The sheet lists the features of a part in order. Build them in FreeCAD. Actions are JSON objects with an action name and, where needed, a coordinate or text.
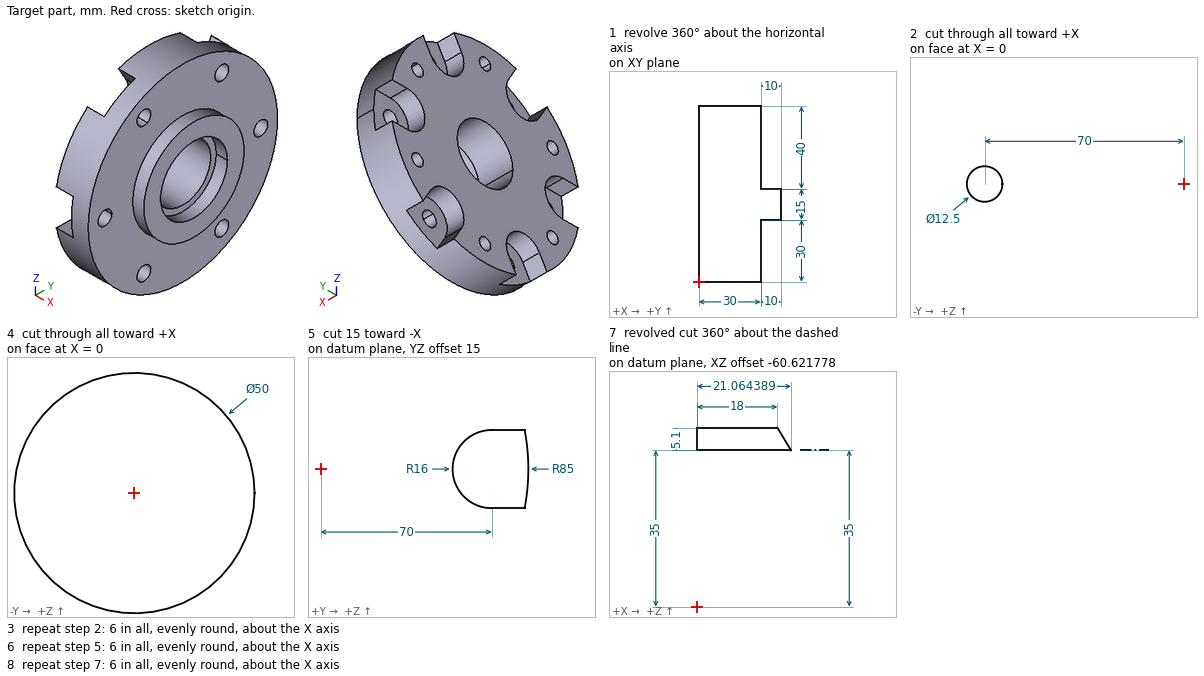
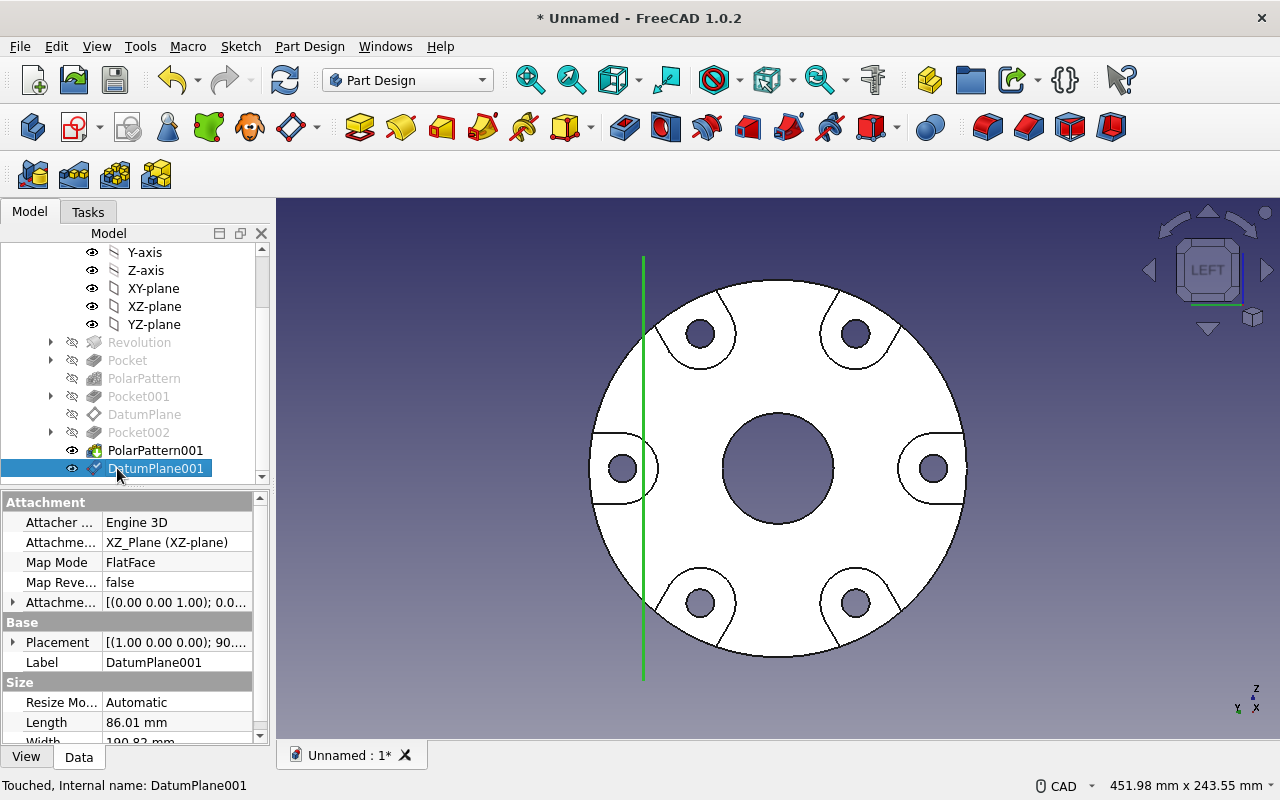
{"action": "left_click", "coordinate": [74, 128]}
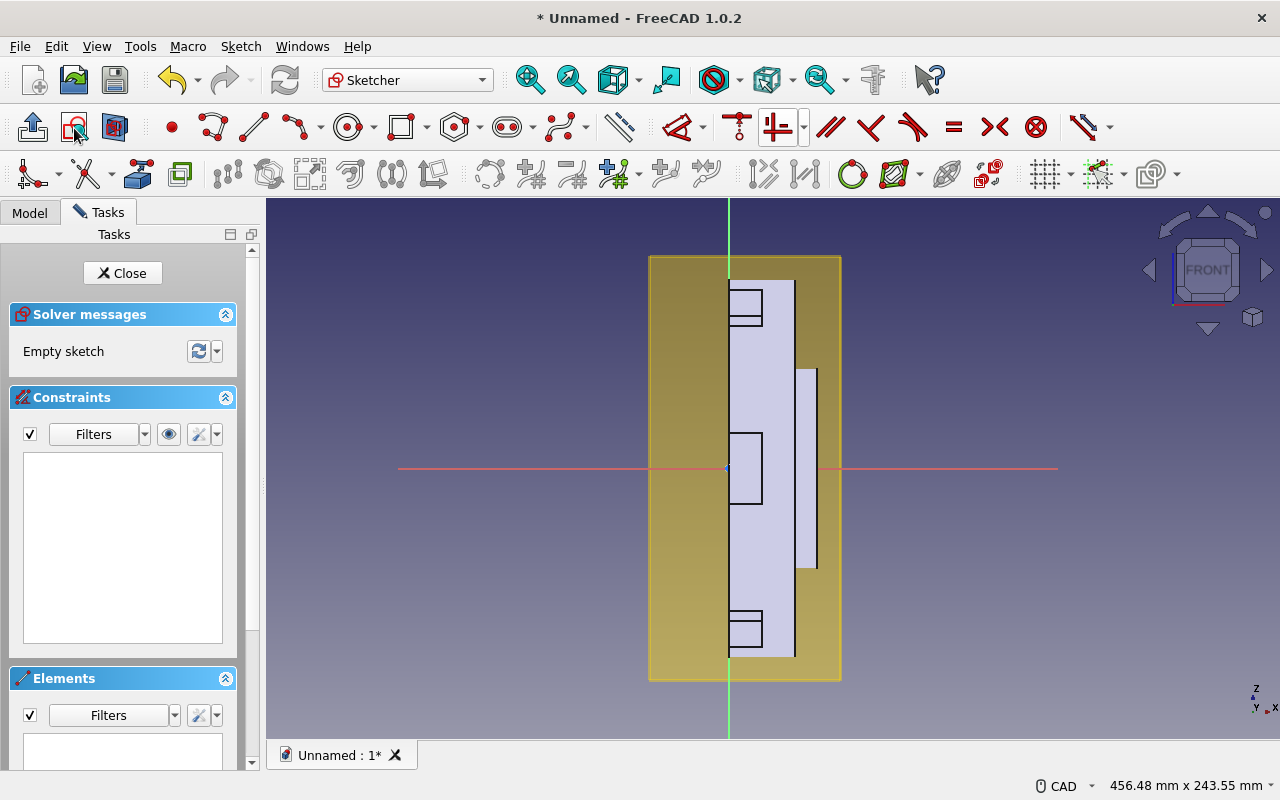
{"action": "left_click", "coordinate": [115, 128]}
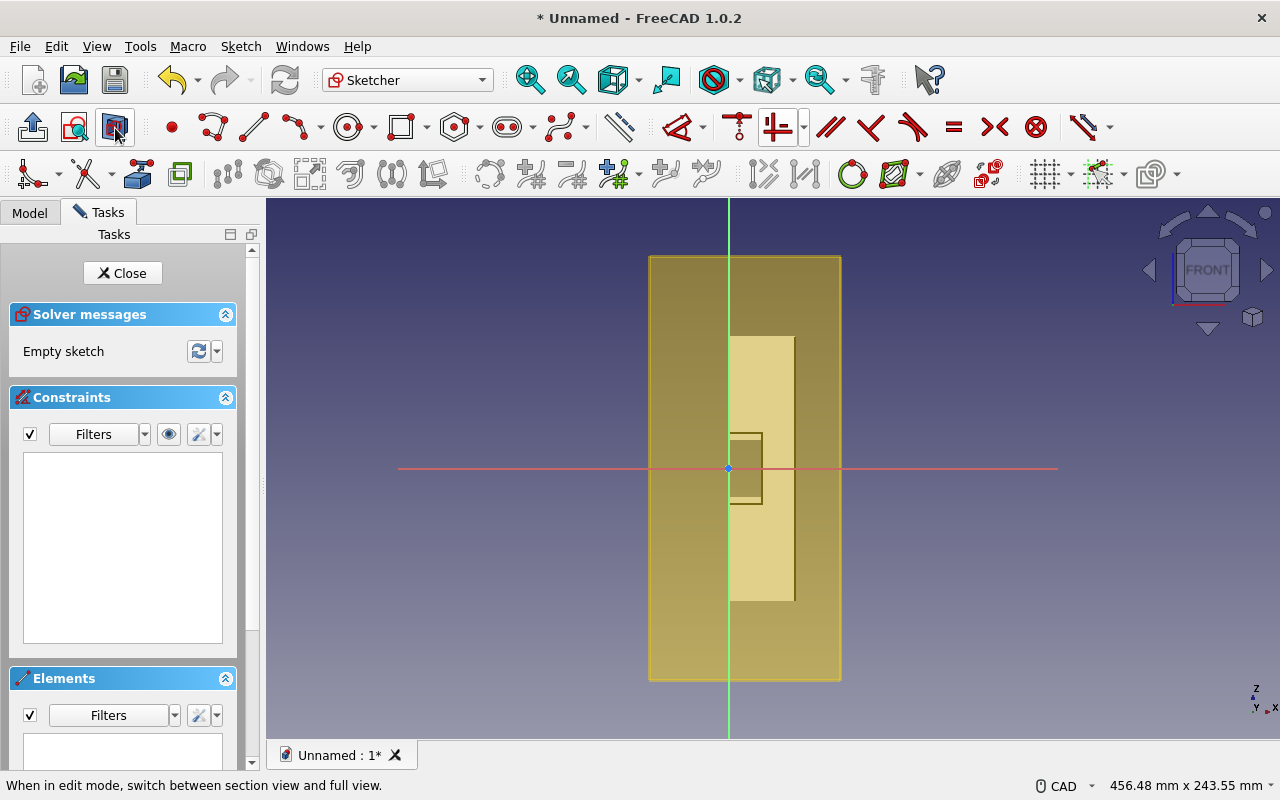
{"action": "scroll", "coordinate": [780, 409], "scroll_direction": "up", "scroll_amount": 7}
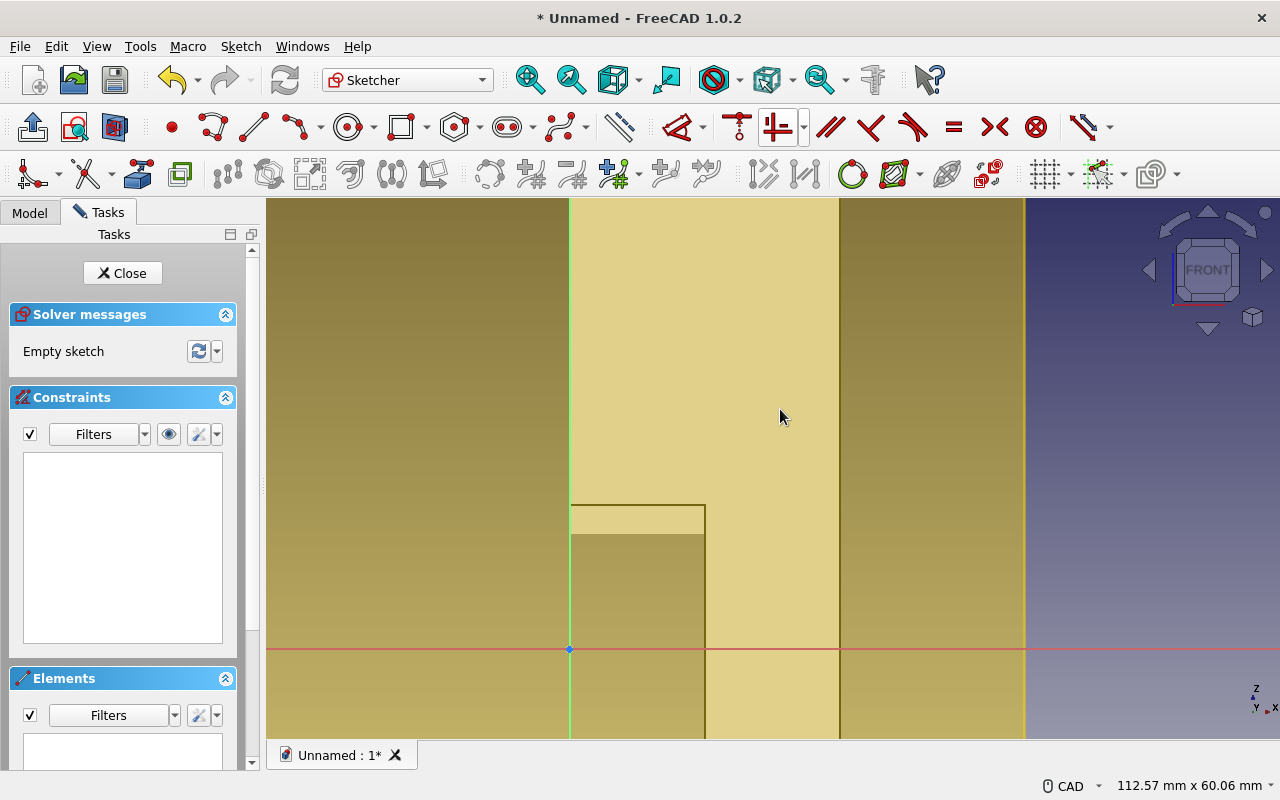
{"action": "left_click", "coordinate": [213, 128]}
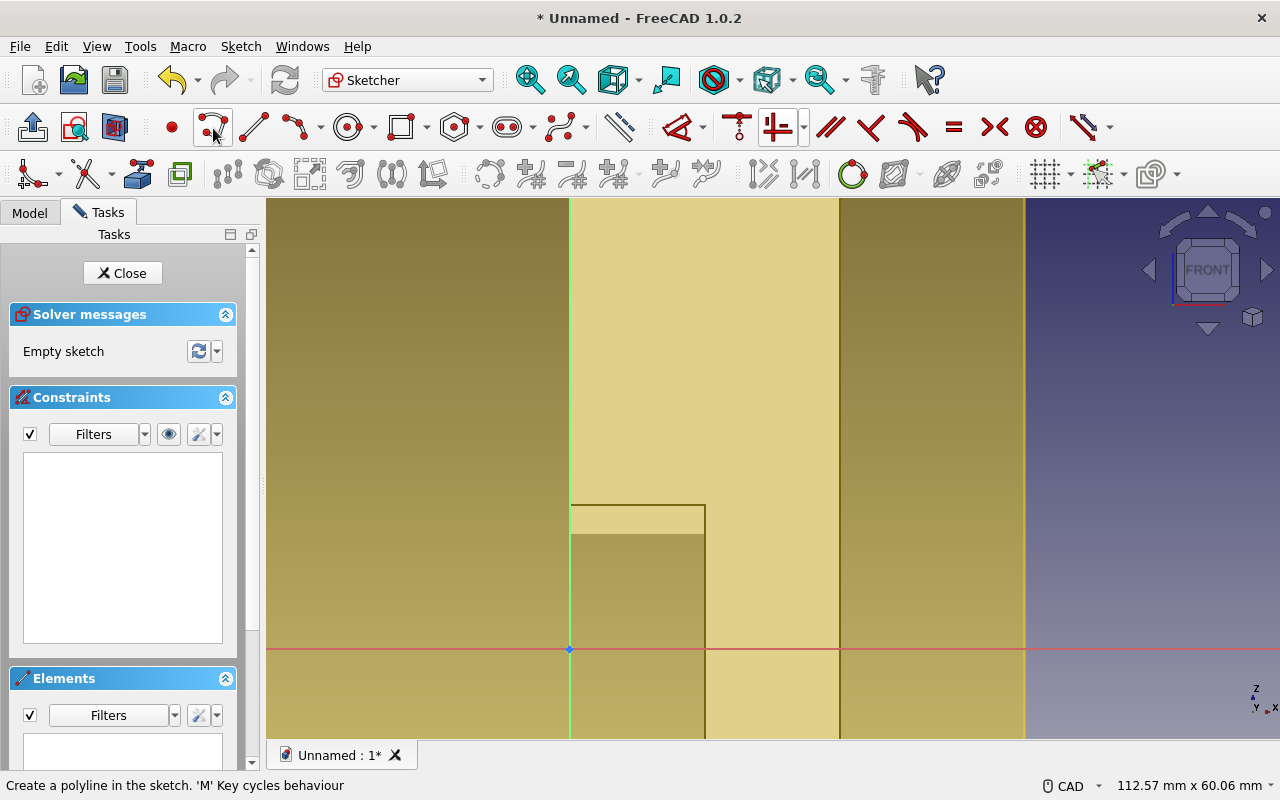
{"action": "left_click", "coordinate": [570, 334]}
{"action": "left_click", "coordinate": [579, 288]}
{"action": "left_click", "coordinate": [732, 288]}
{"action": "left_click", "coordinate": [760, 334]}
{"action": "left_click", "coordinate": [570, 335]}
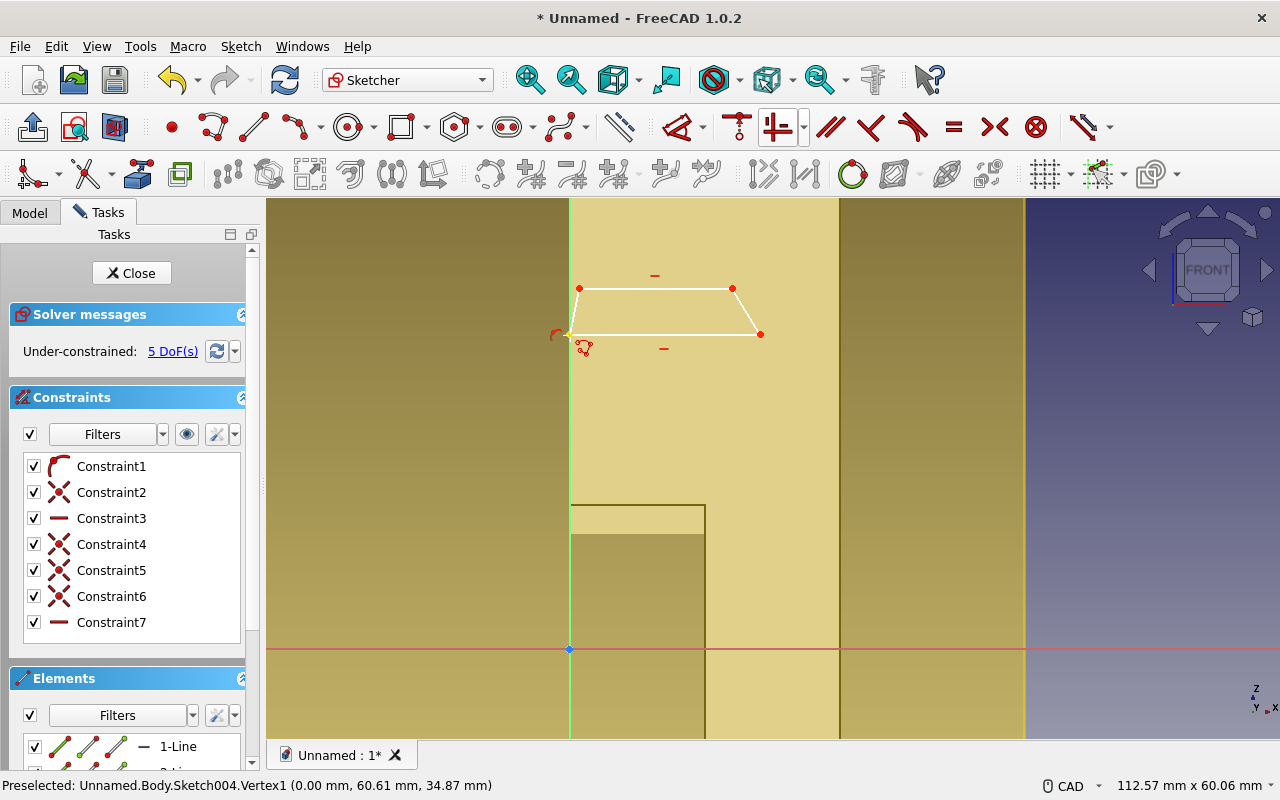
{"action": "left_click", "coordinate": [254, 128]}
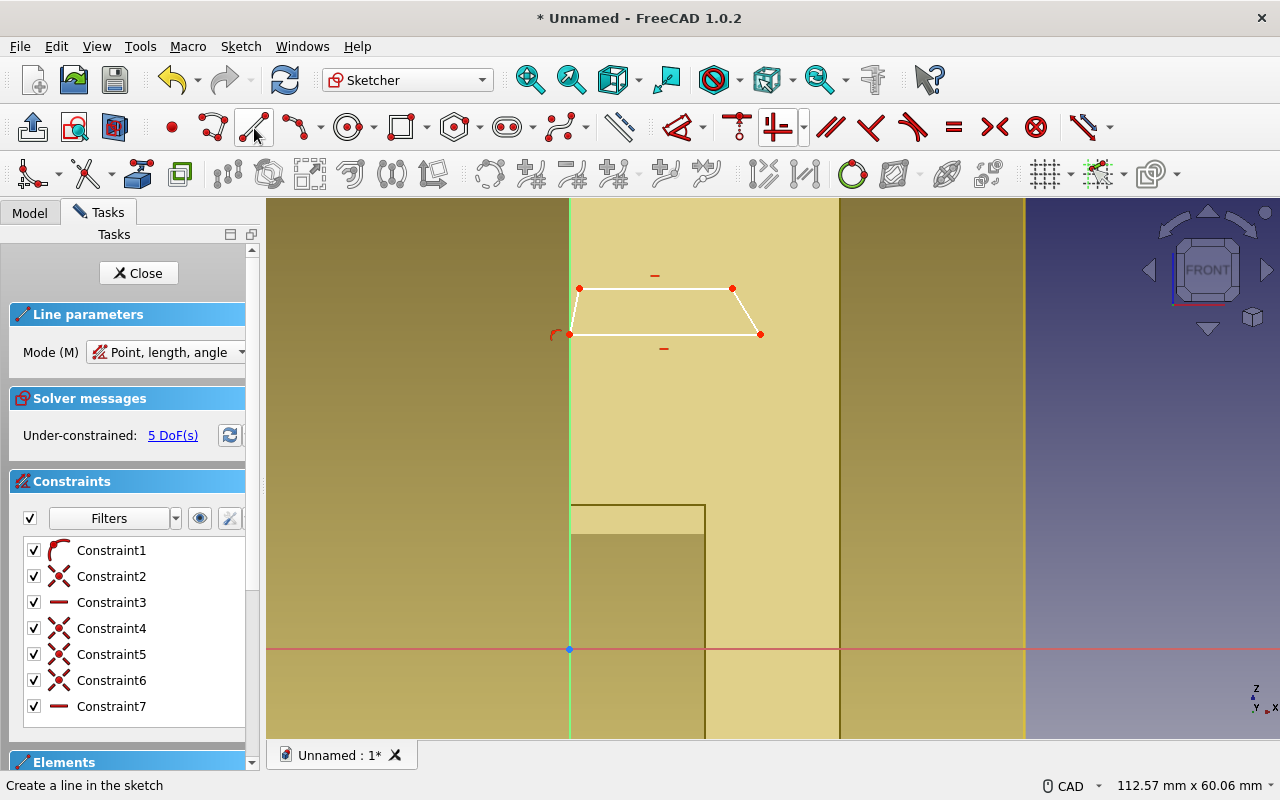
{"action": "left_click", "coordinate": [779, 334]}
{"action": "left_click", "coordinate": [836, 334]}
{"action": "key", "text": "Escape"}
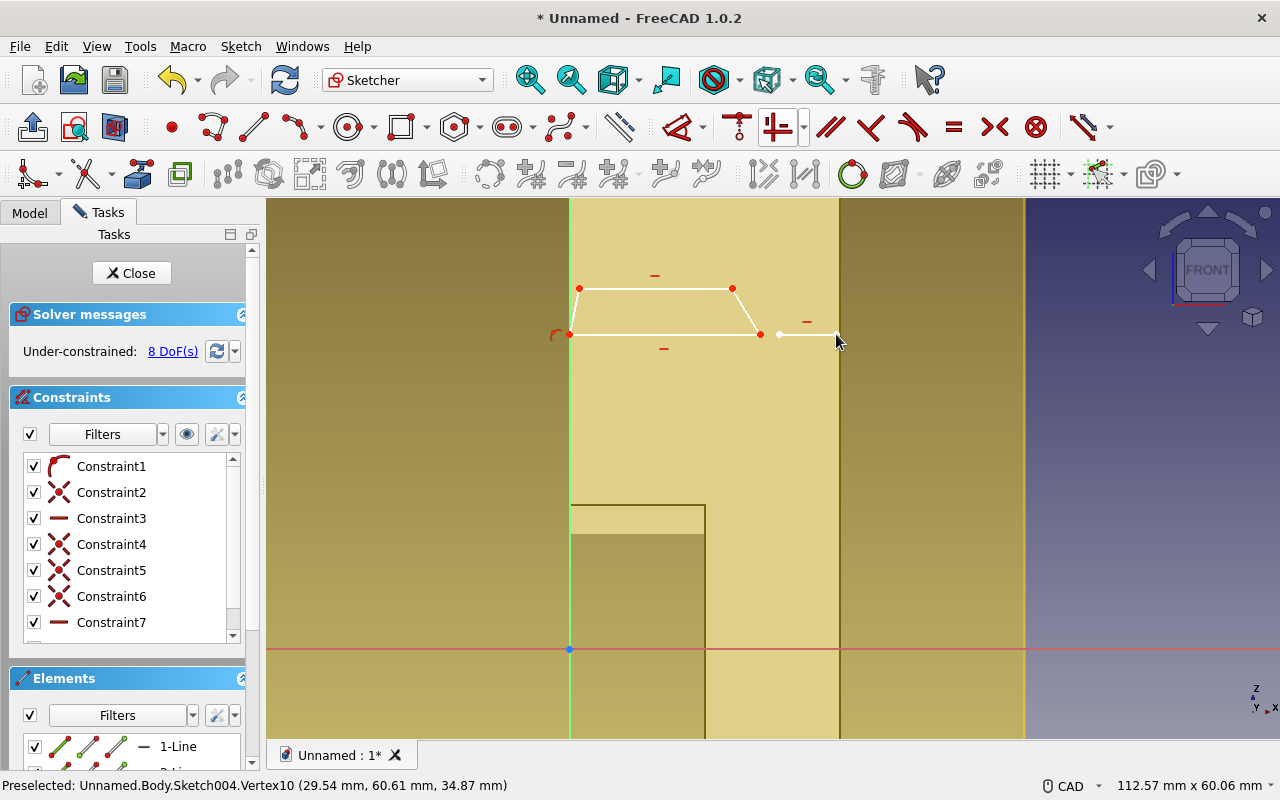
{"action": "left_click", "coordinate": [796, 335]}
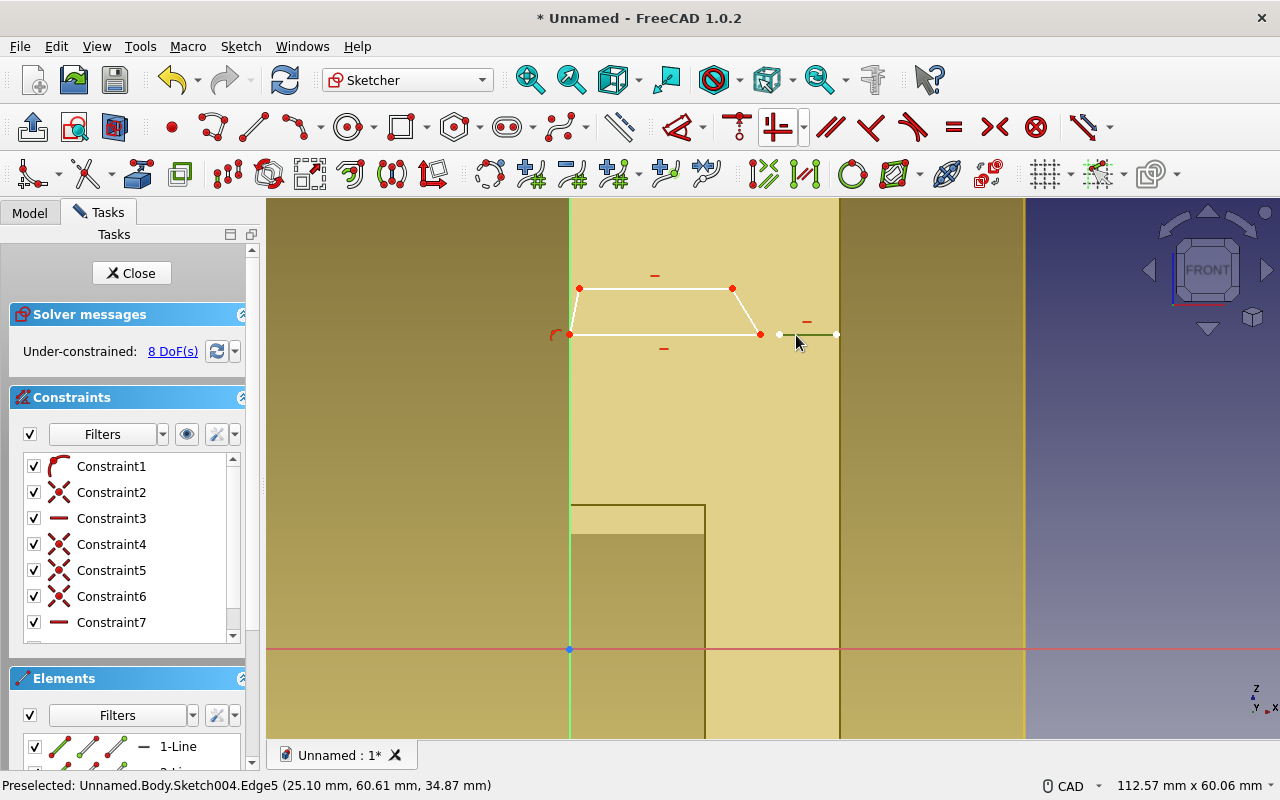
{"action": "left_click", "coordinate": [620, 128]}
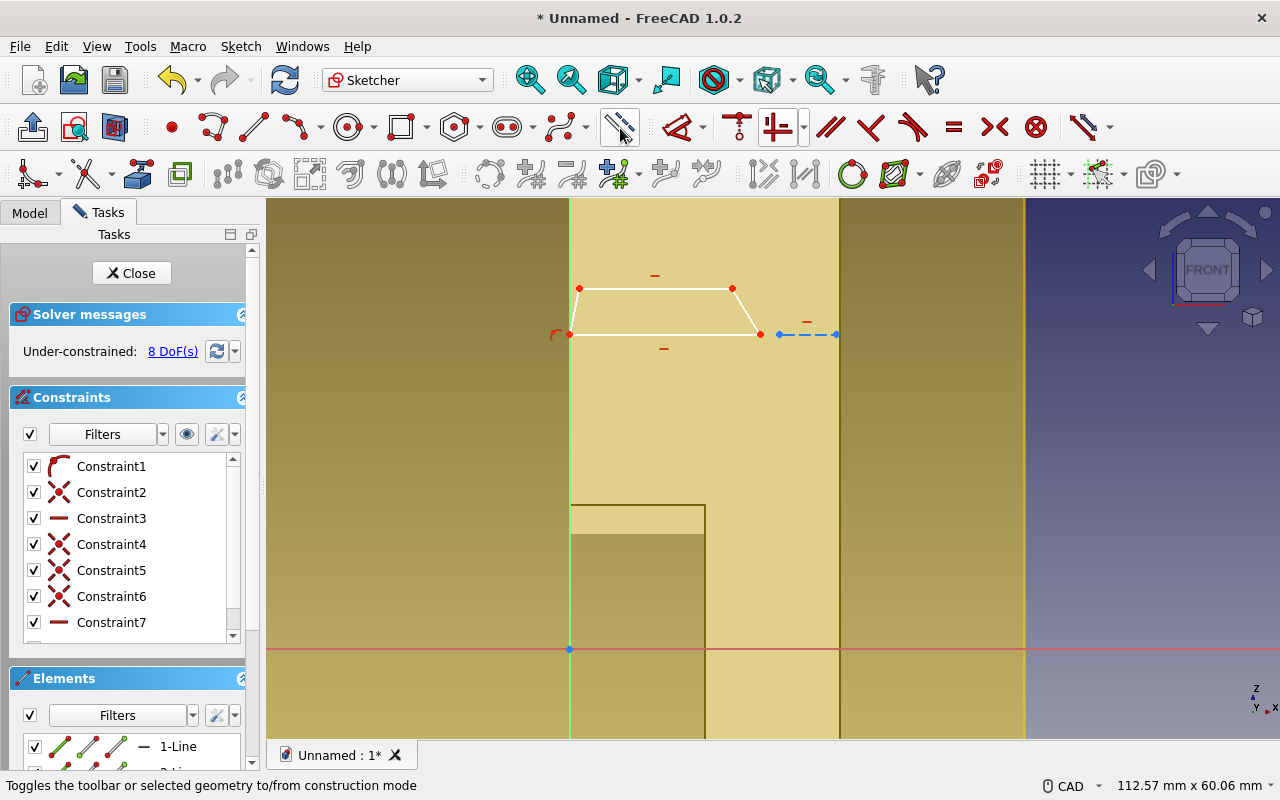
{"action": "left_click", "coordinate": [573, 321]}